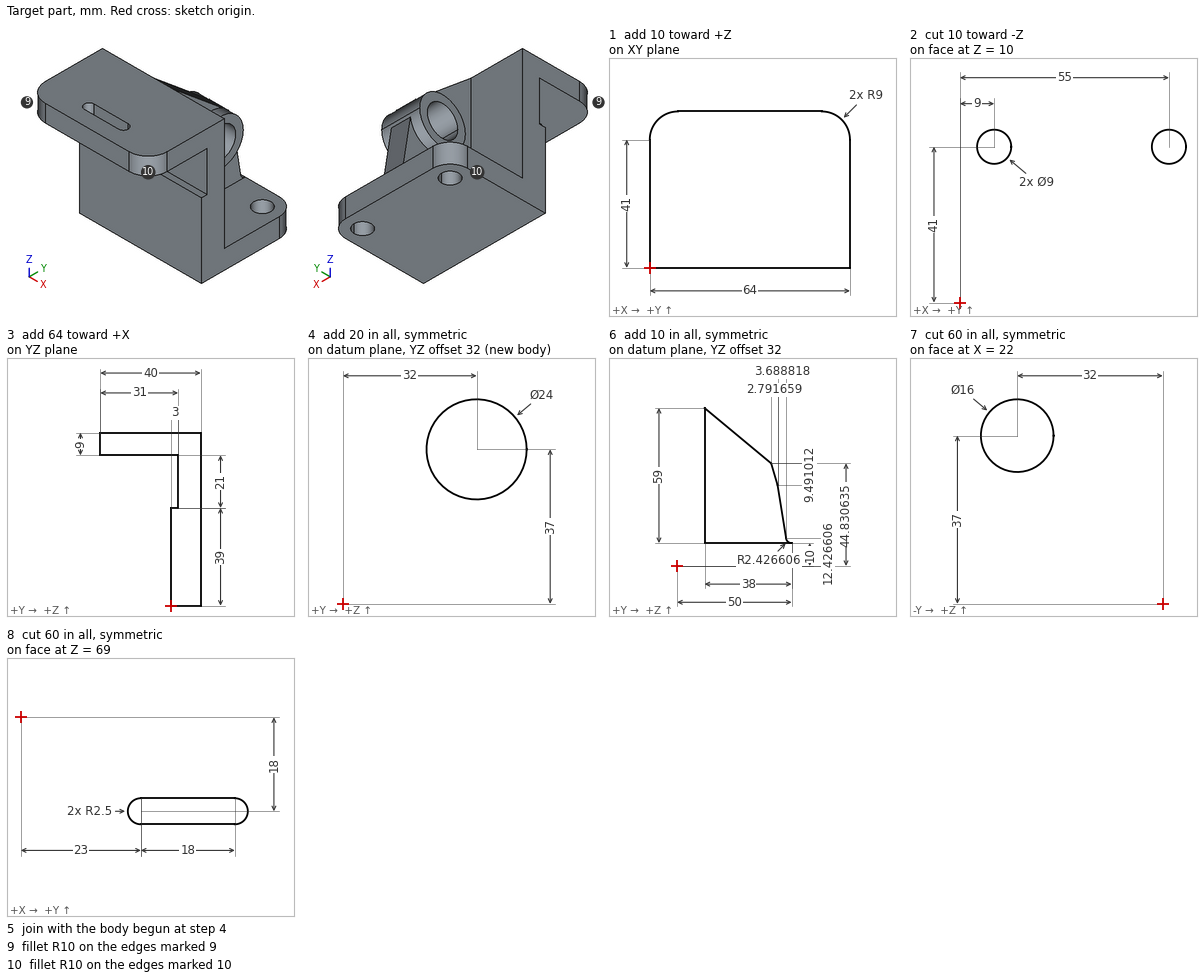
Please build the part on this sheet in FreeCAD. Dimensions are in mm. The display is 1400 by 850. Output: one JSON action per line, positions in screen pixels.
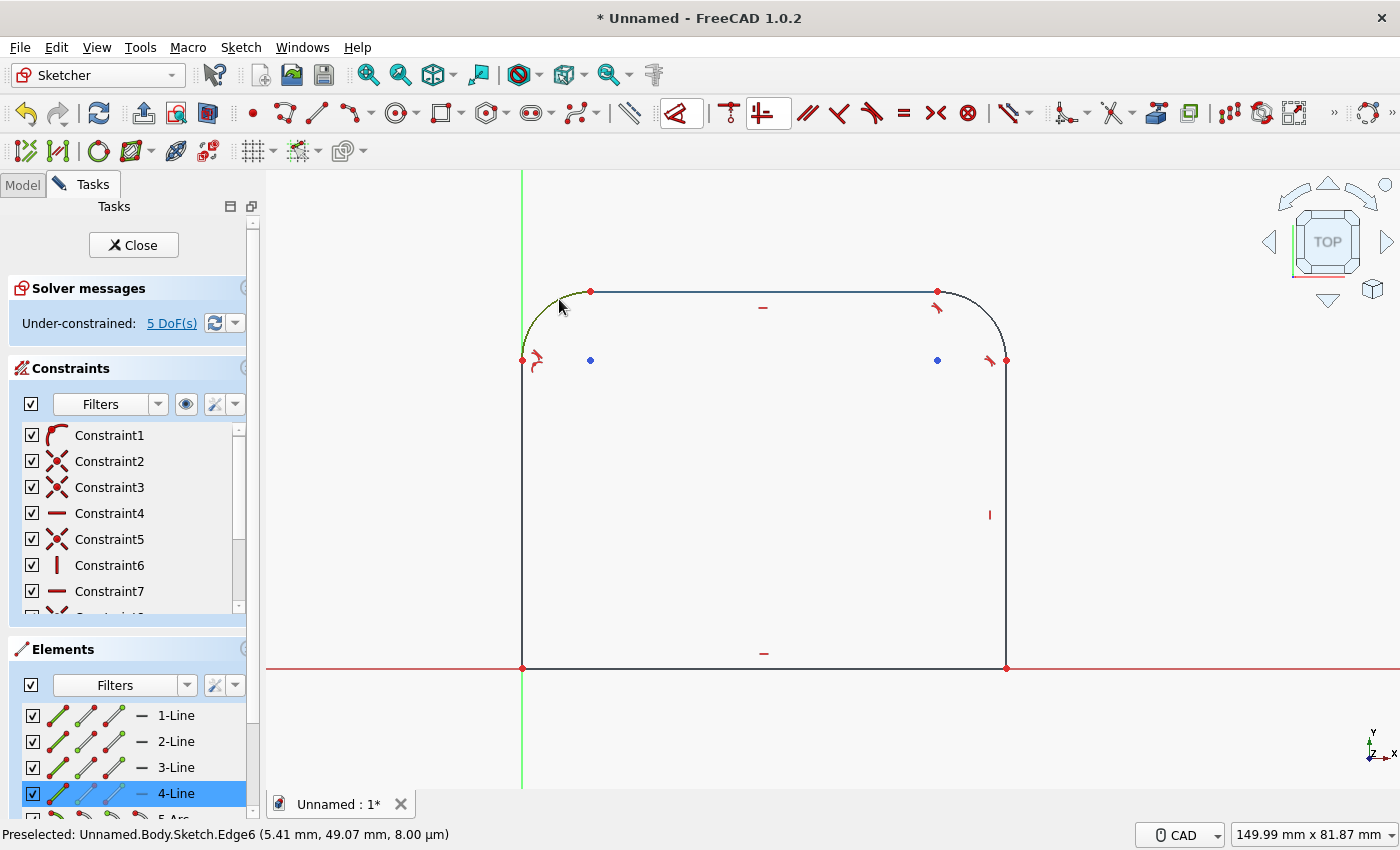
{"action": "left_click", "coordinate": [872, 114]}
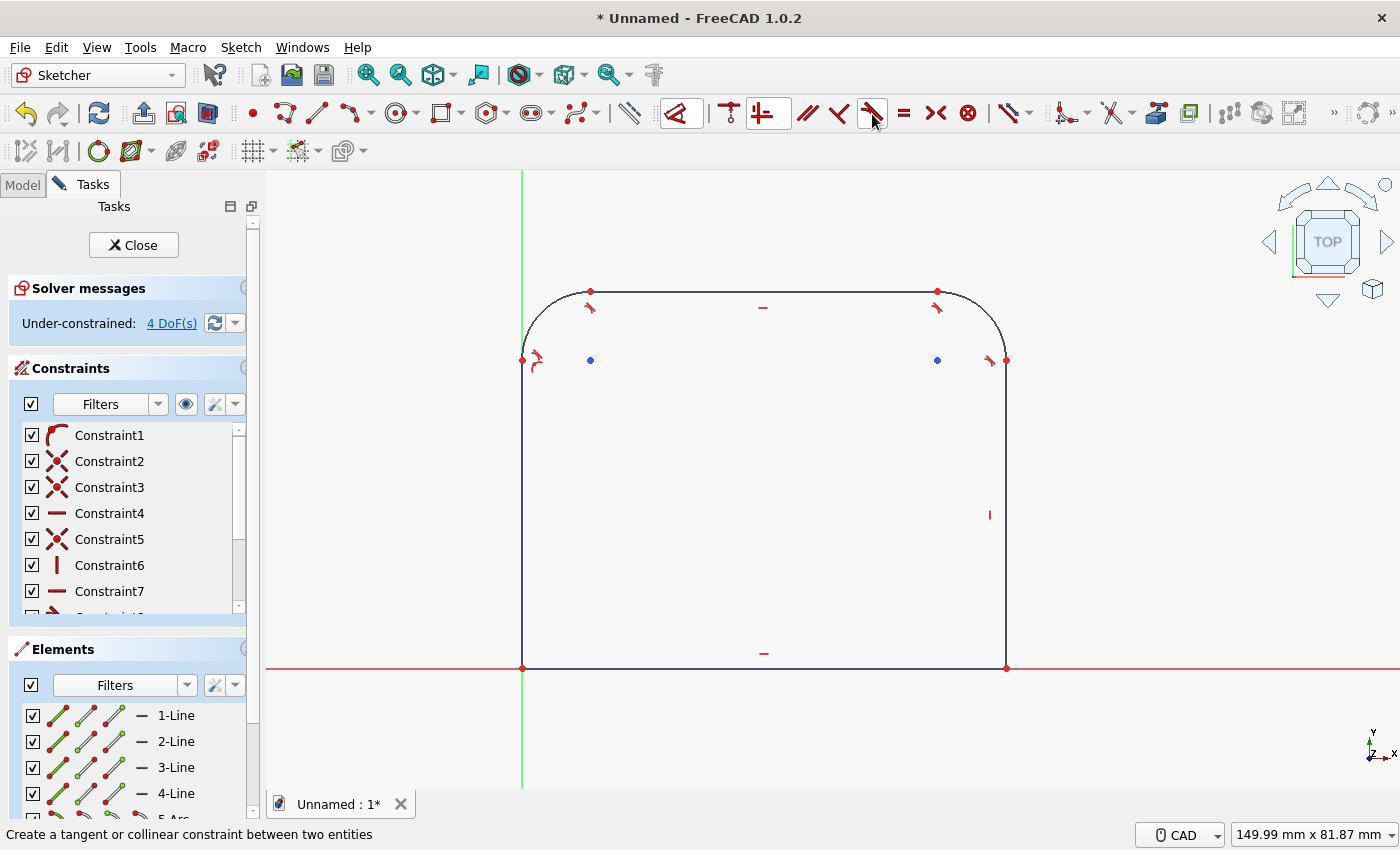
{"action": "left_click", "coordinate": [999, 329]}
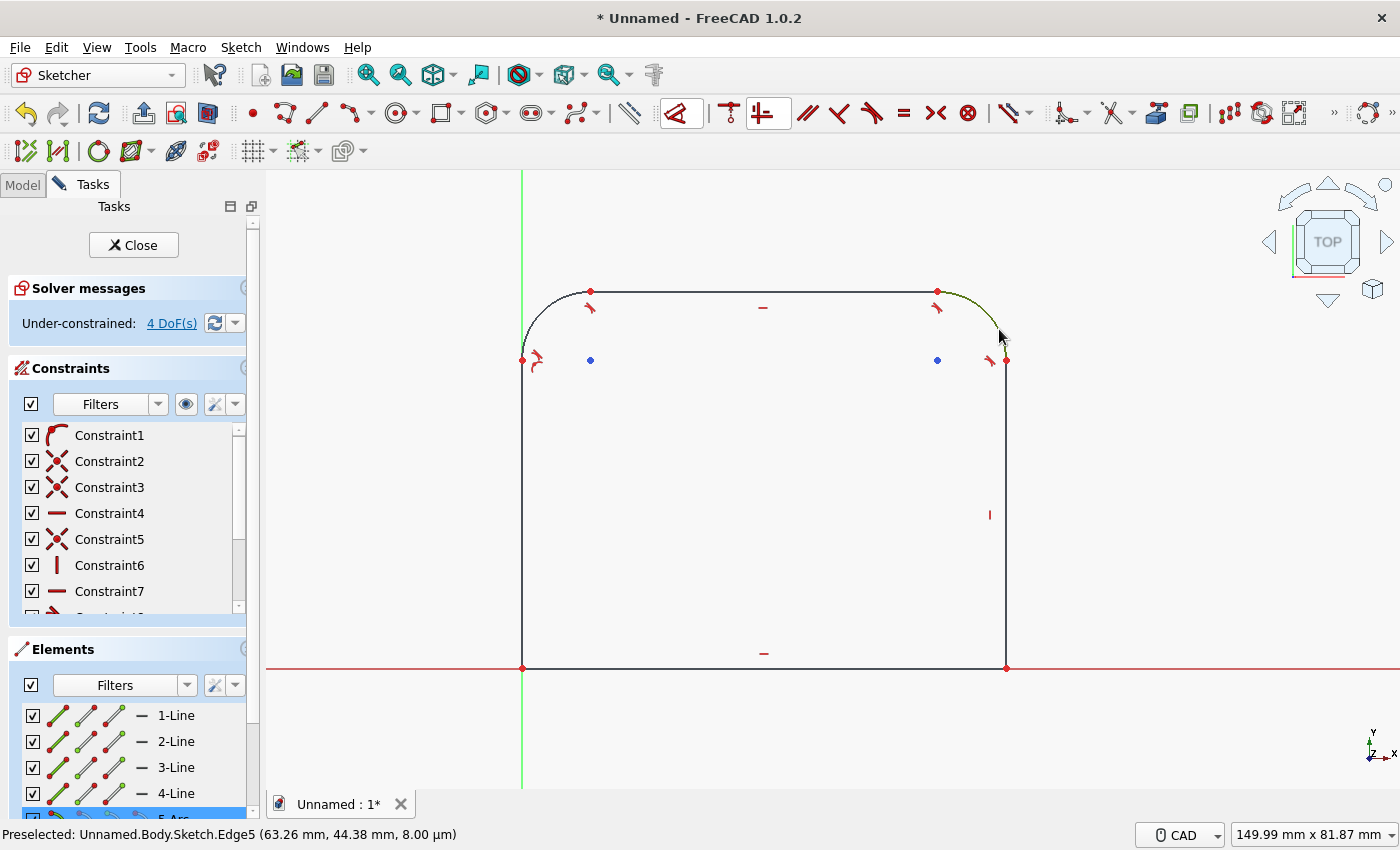
{"action": "left_click", "coordinate": [559, 299]}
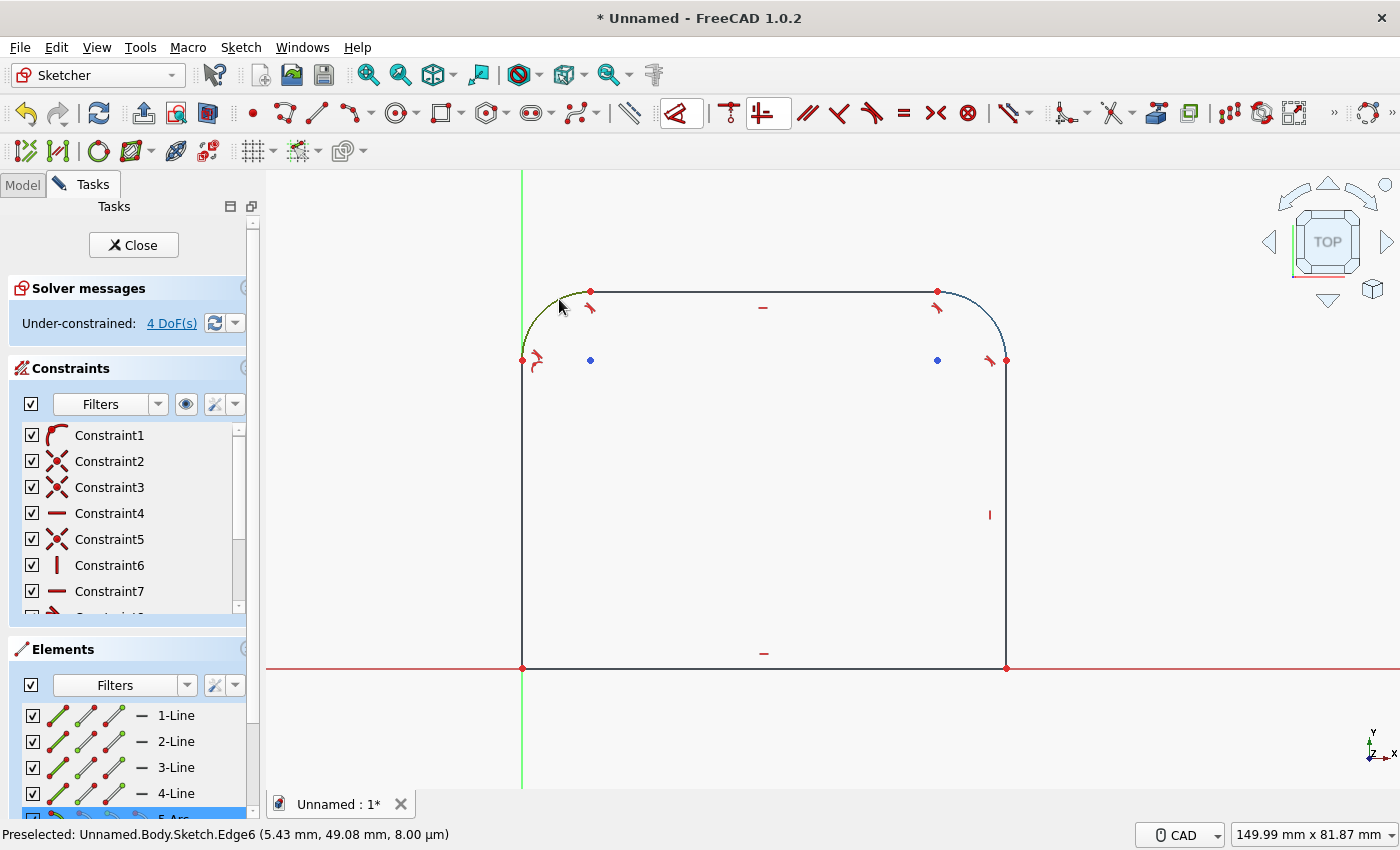
{"action": "left_click", "coordinate": [904, 114]}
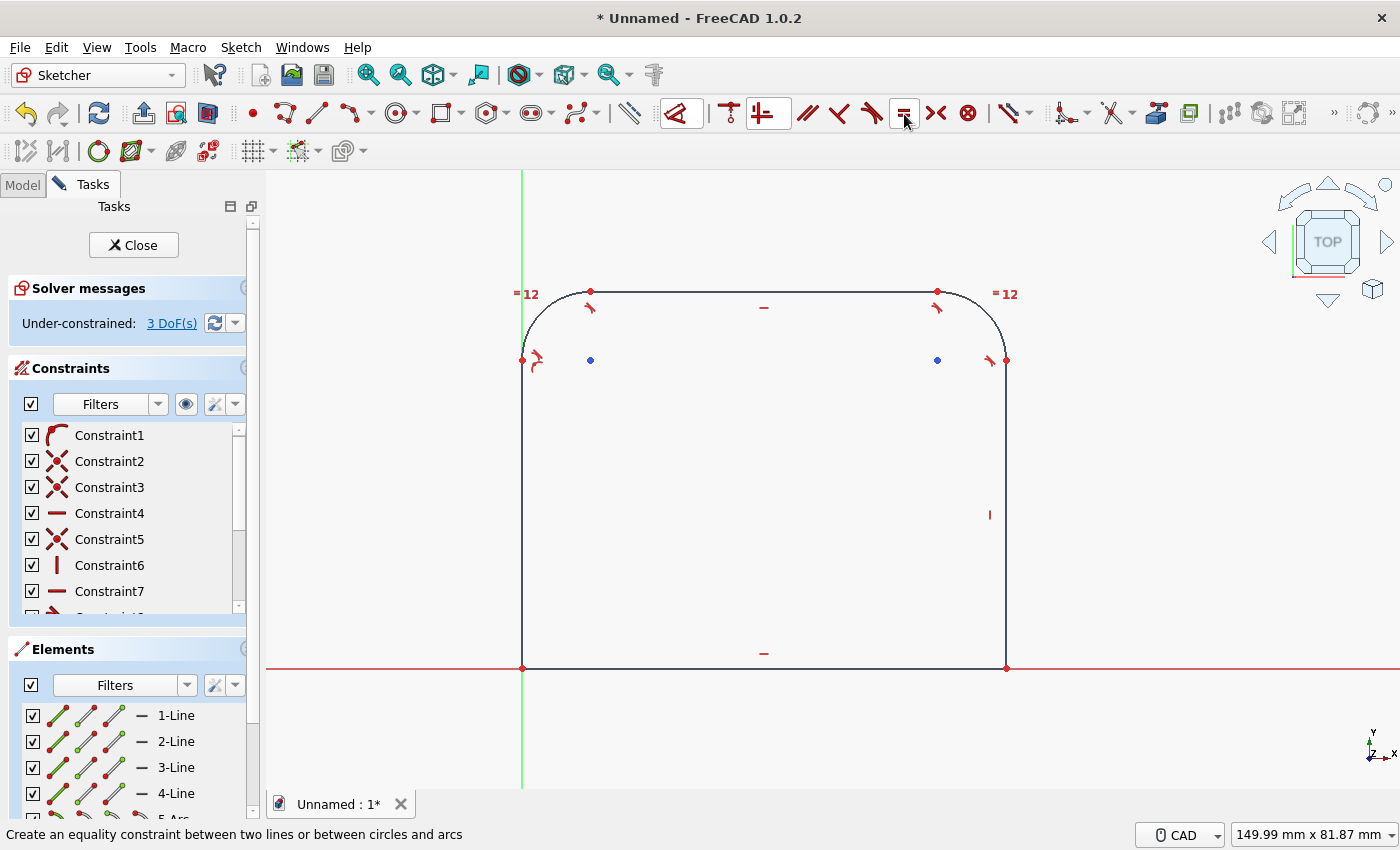
{"action": "left_click", "coordinate": [676, 114]}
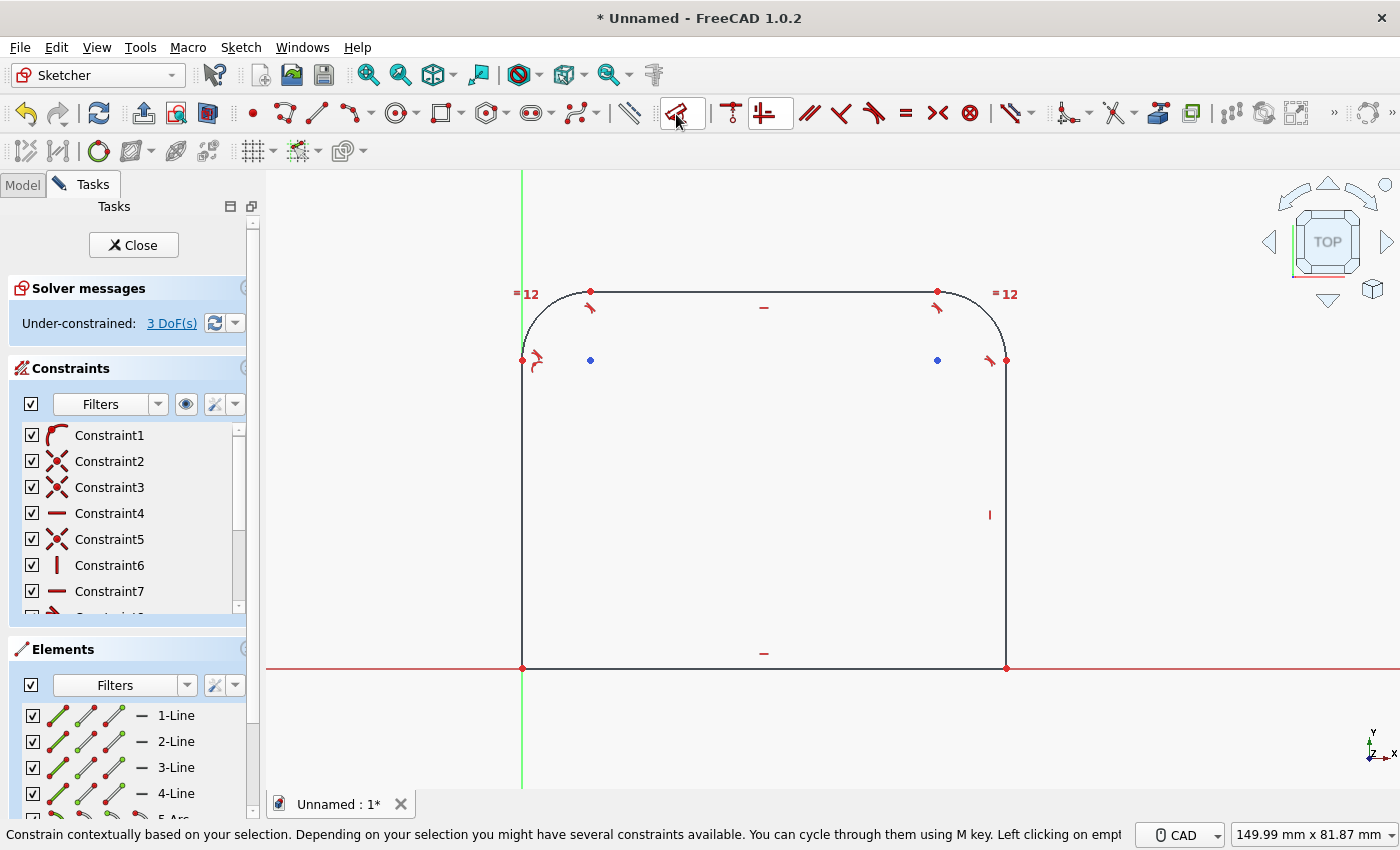
{"action": "left_click", "coordinate": [999, 329]}
{"action": "left_click", "coordinate": [1028, 314]}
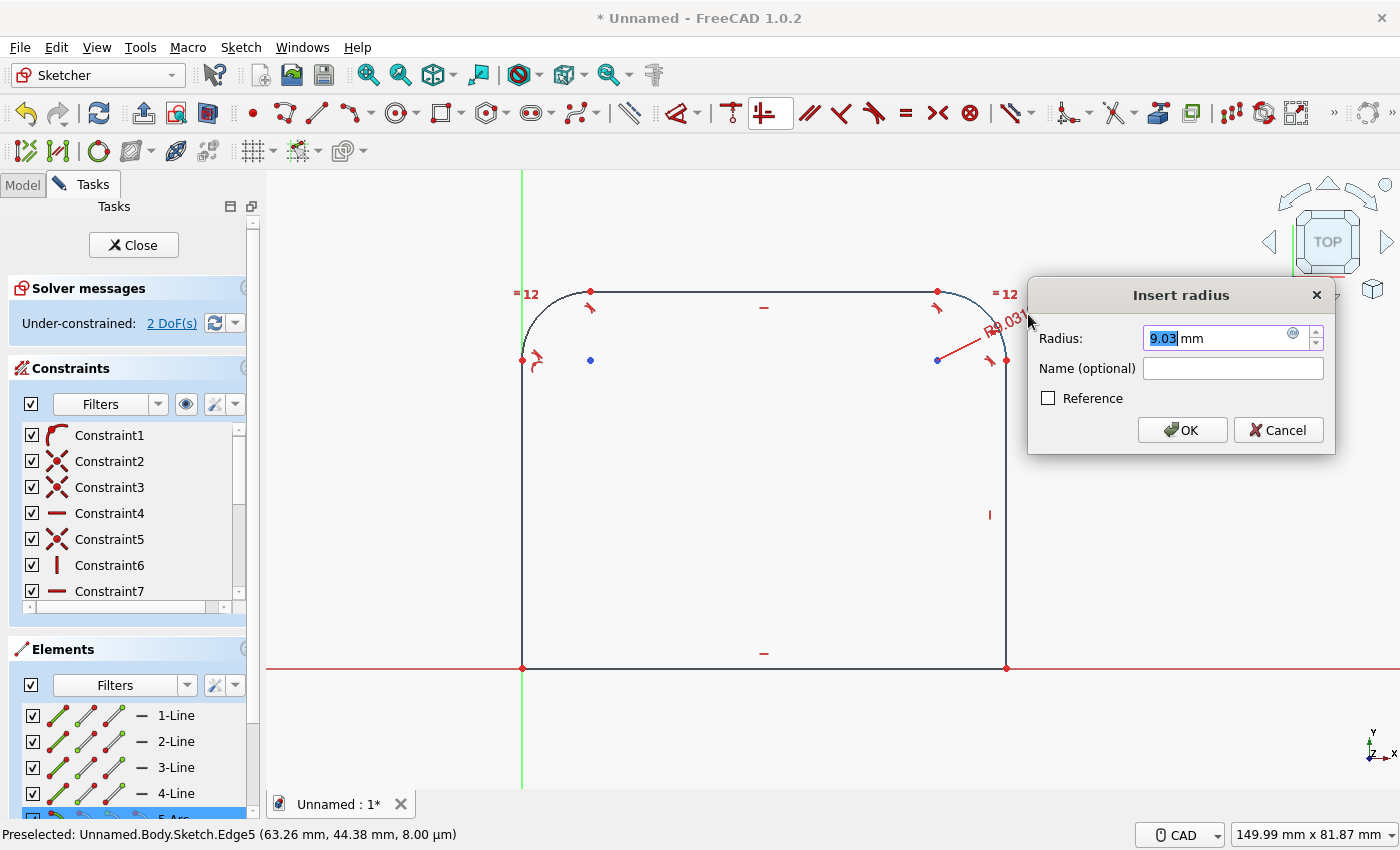
{"action": "type", "text": "9"}
{"action": "key", "text": "Return"}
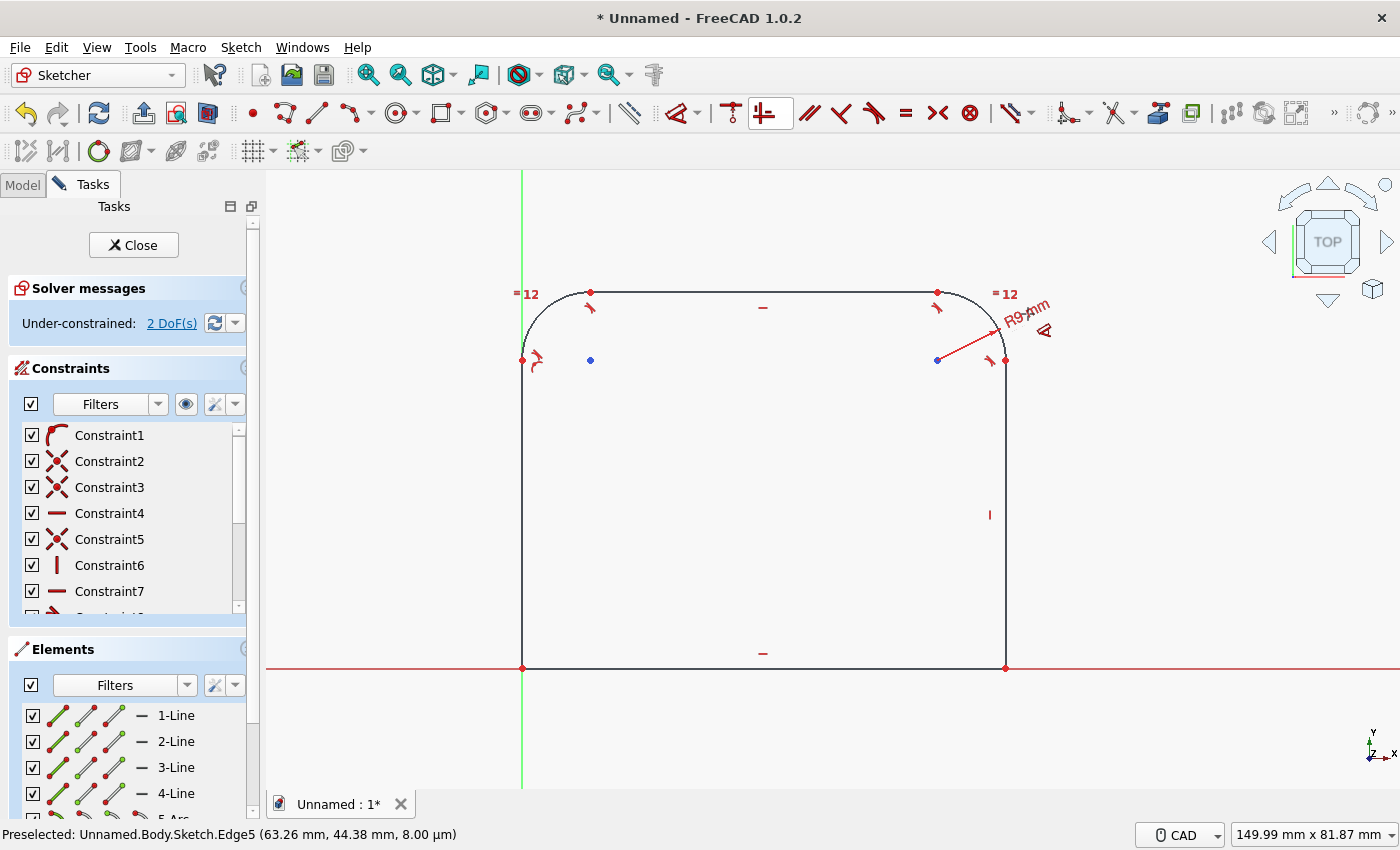
{"action": "left_click", "coordinate": [522, 453]}
{"action": "left_click", "coordinate": [488, 514]}